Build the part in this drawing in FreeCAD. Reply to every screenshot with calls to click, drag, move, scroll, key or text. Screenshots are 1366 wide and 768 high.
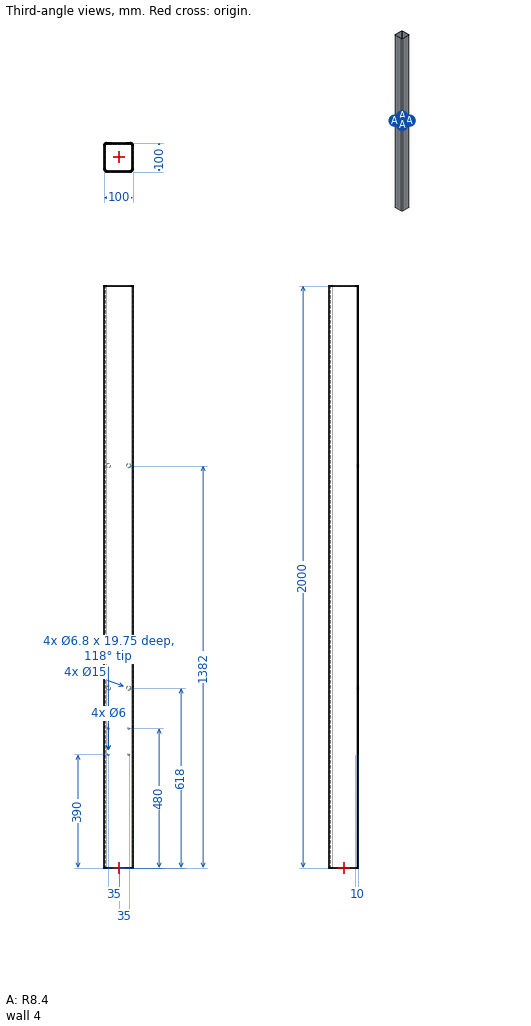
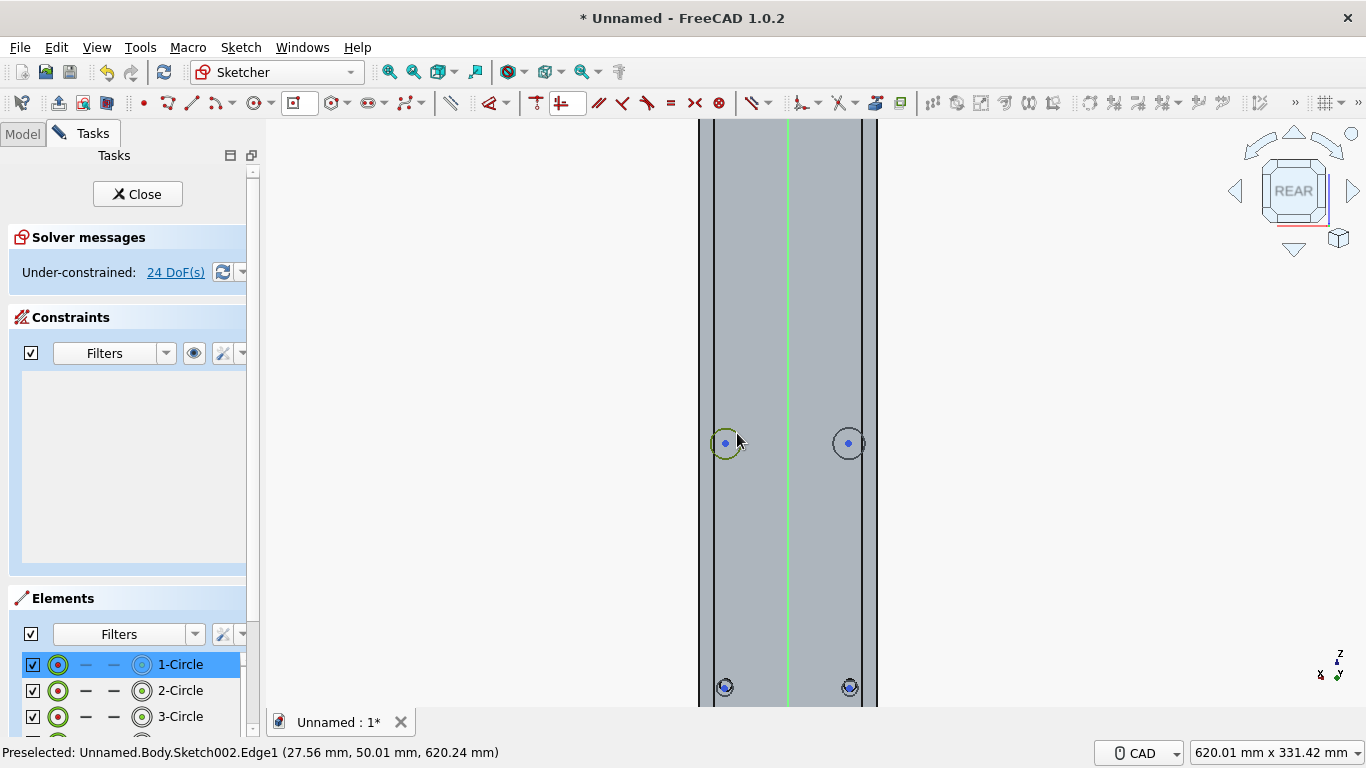
click(860, 432)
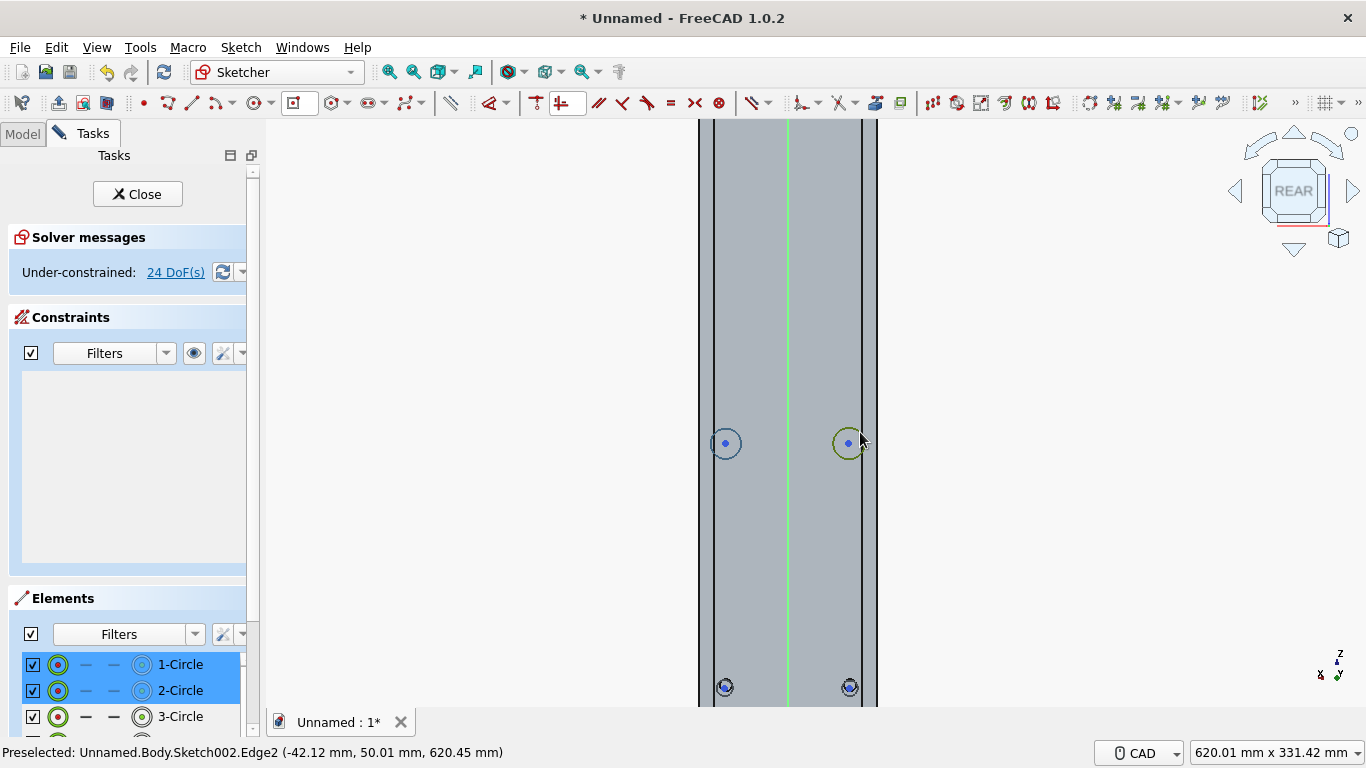
scroll(739, 435, down, 9)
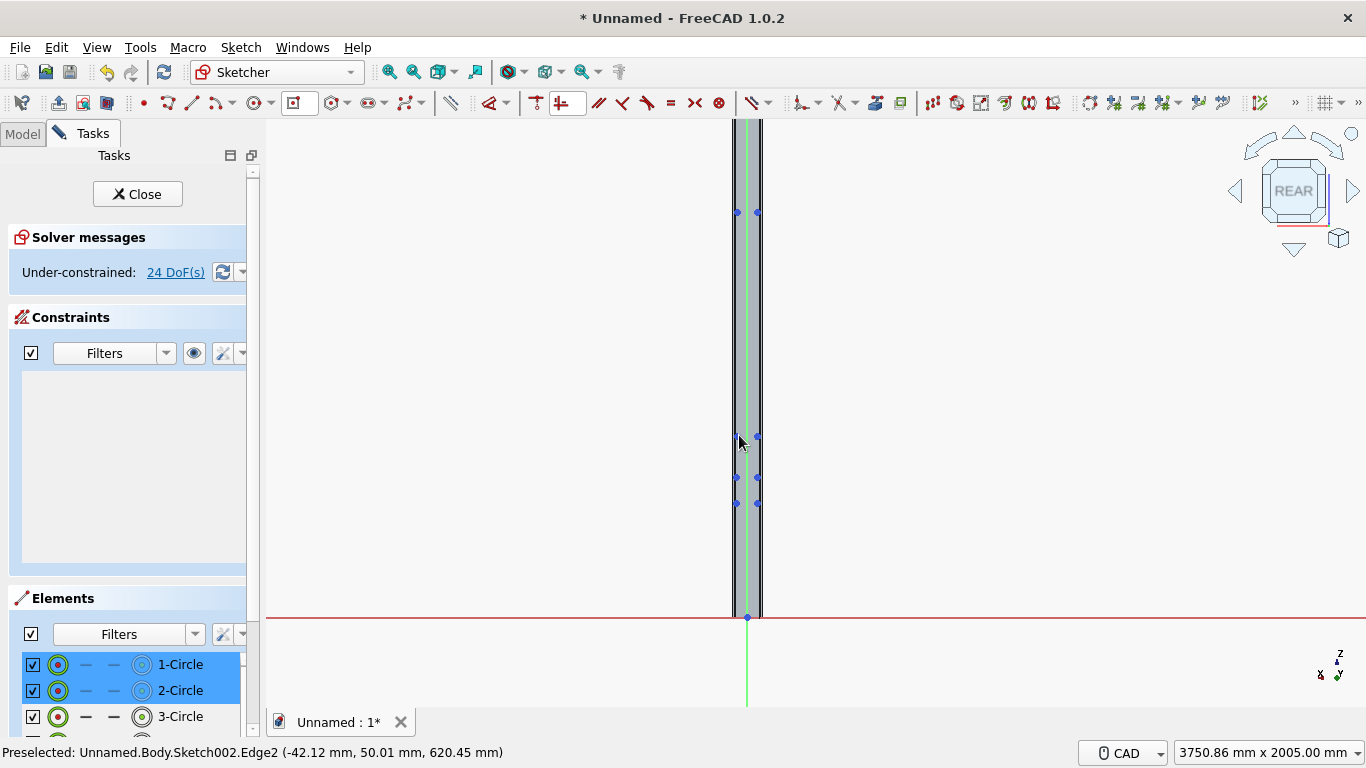
scroll(739, 211, up, 10)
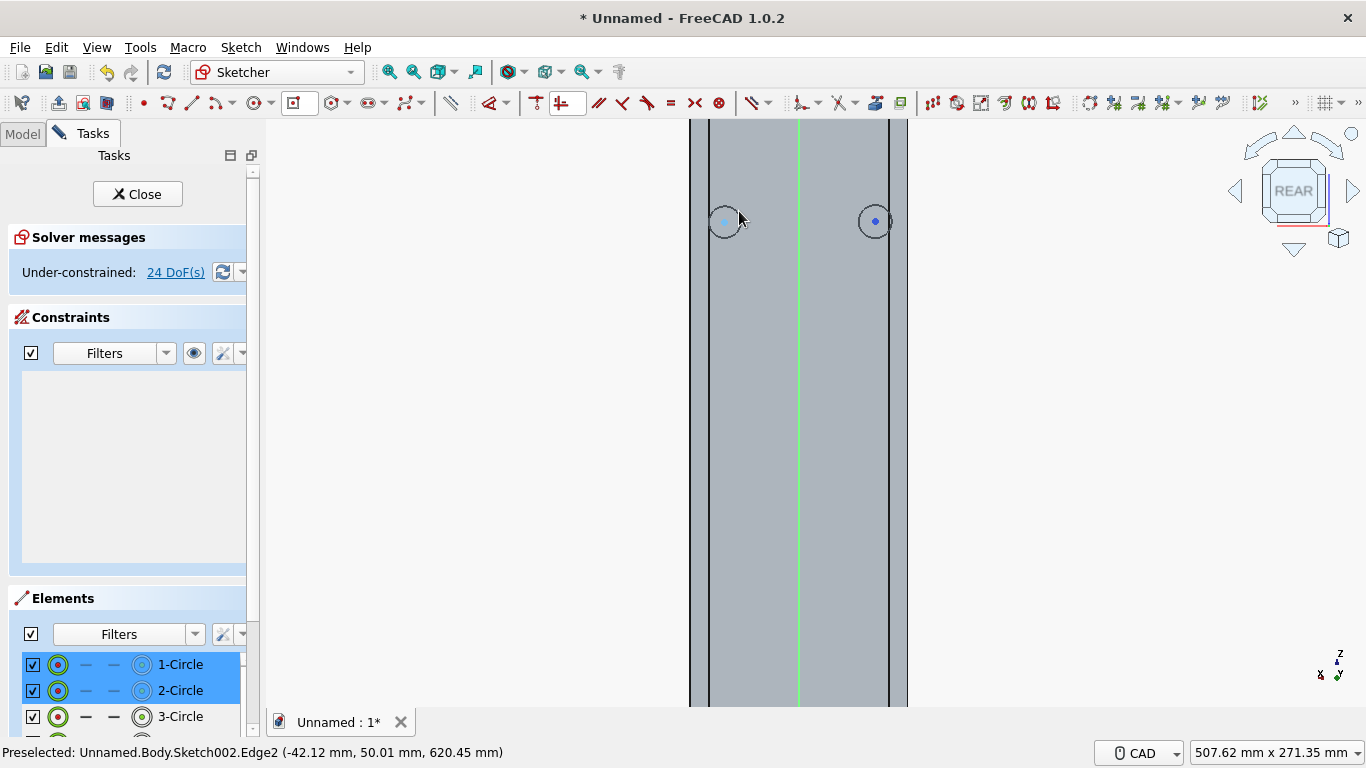
click(736, 211)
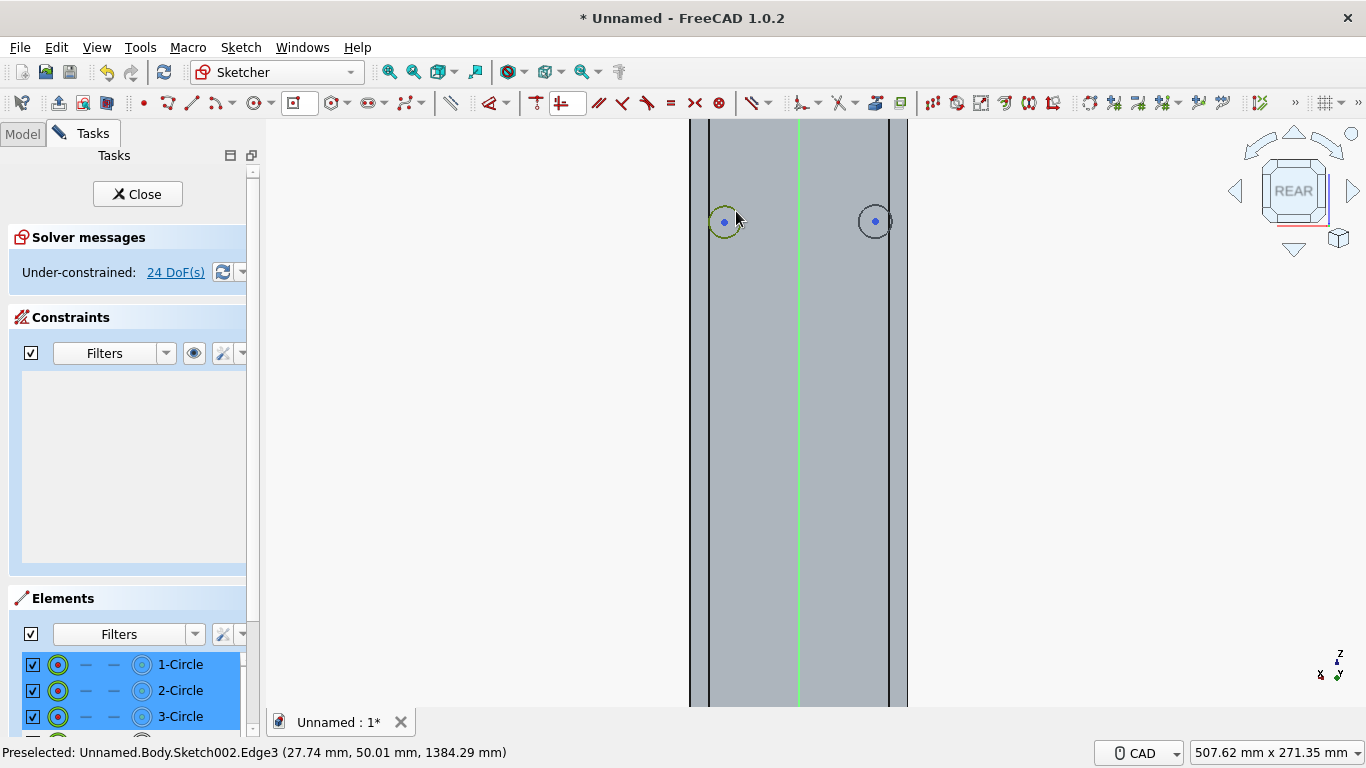
click(887, 210)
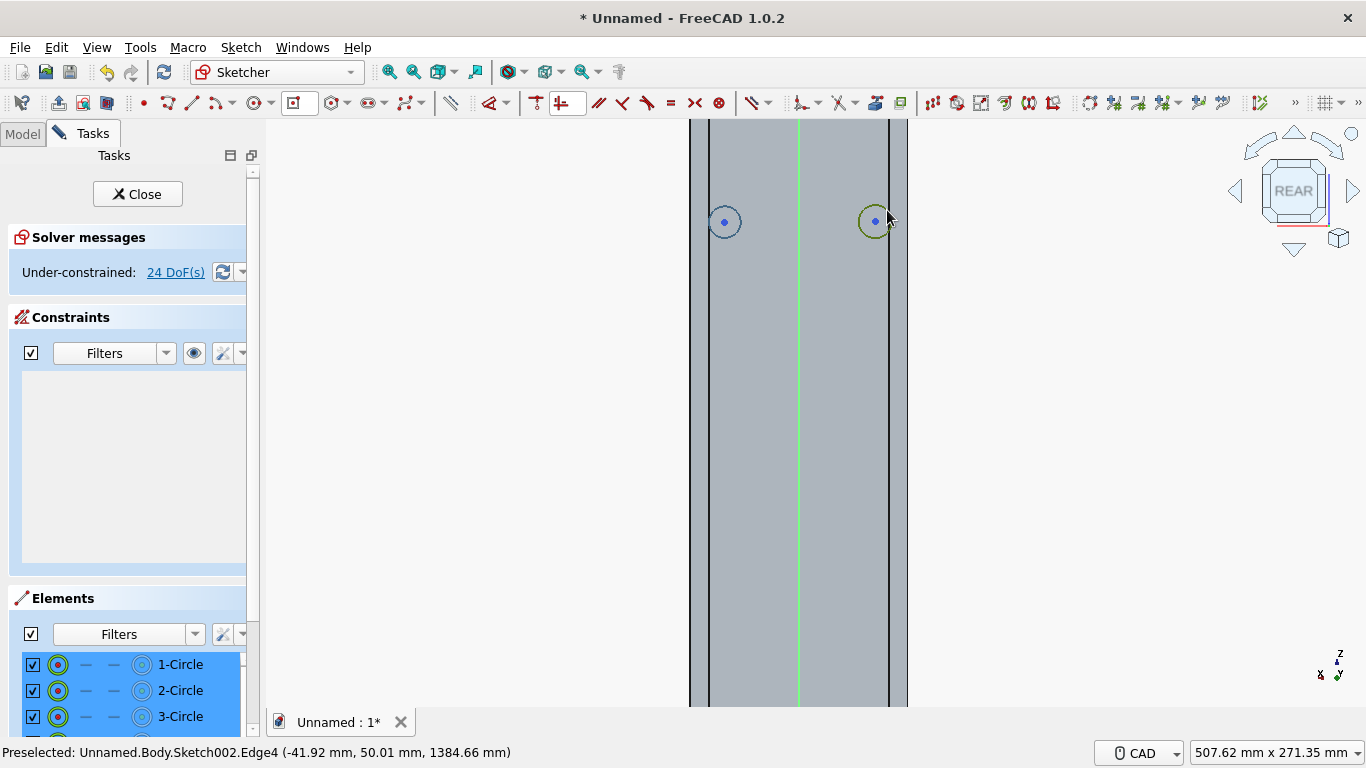
click(672, 104)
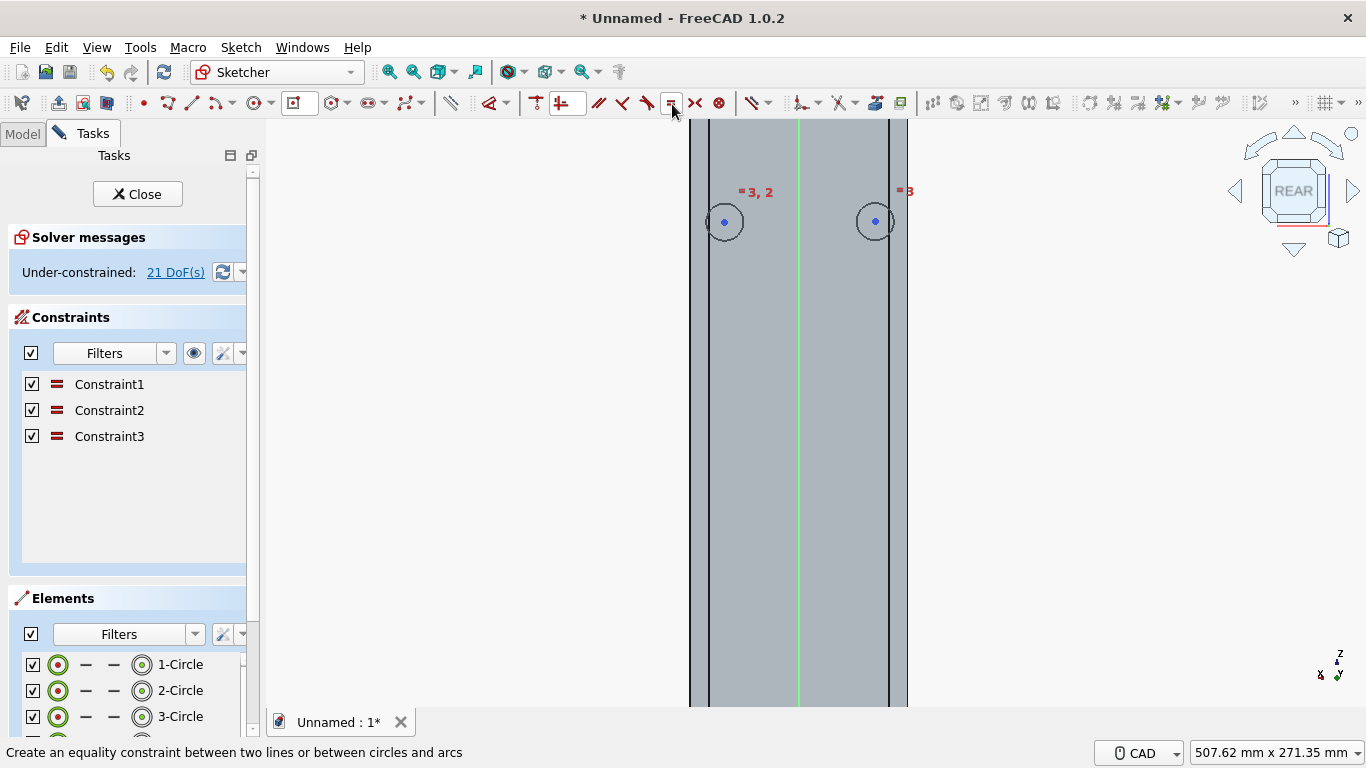
scroll(739, 210, down, 10)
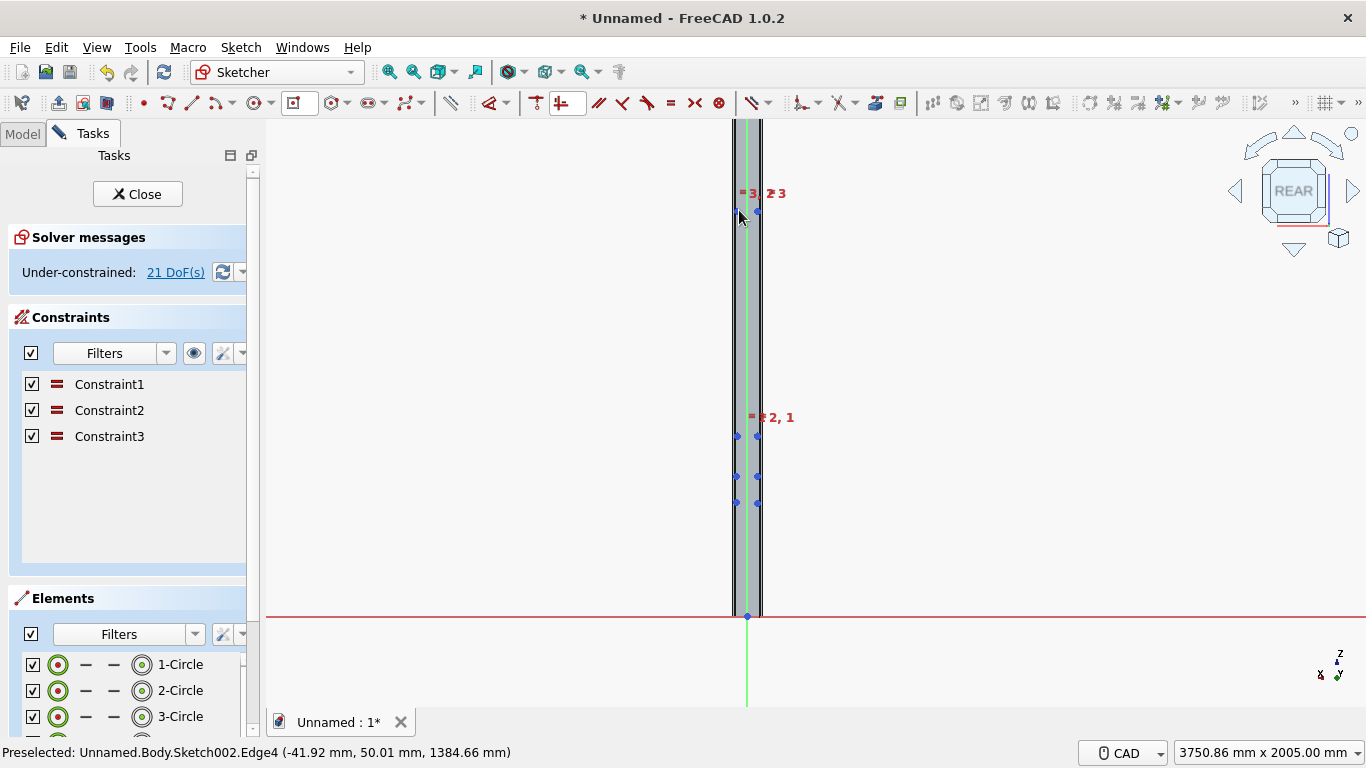
scroll(759, 502, up, 12)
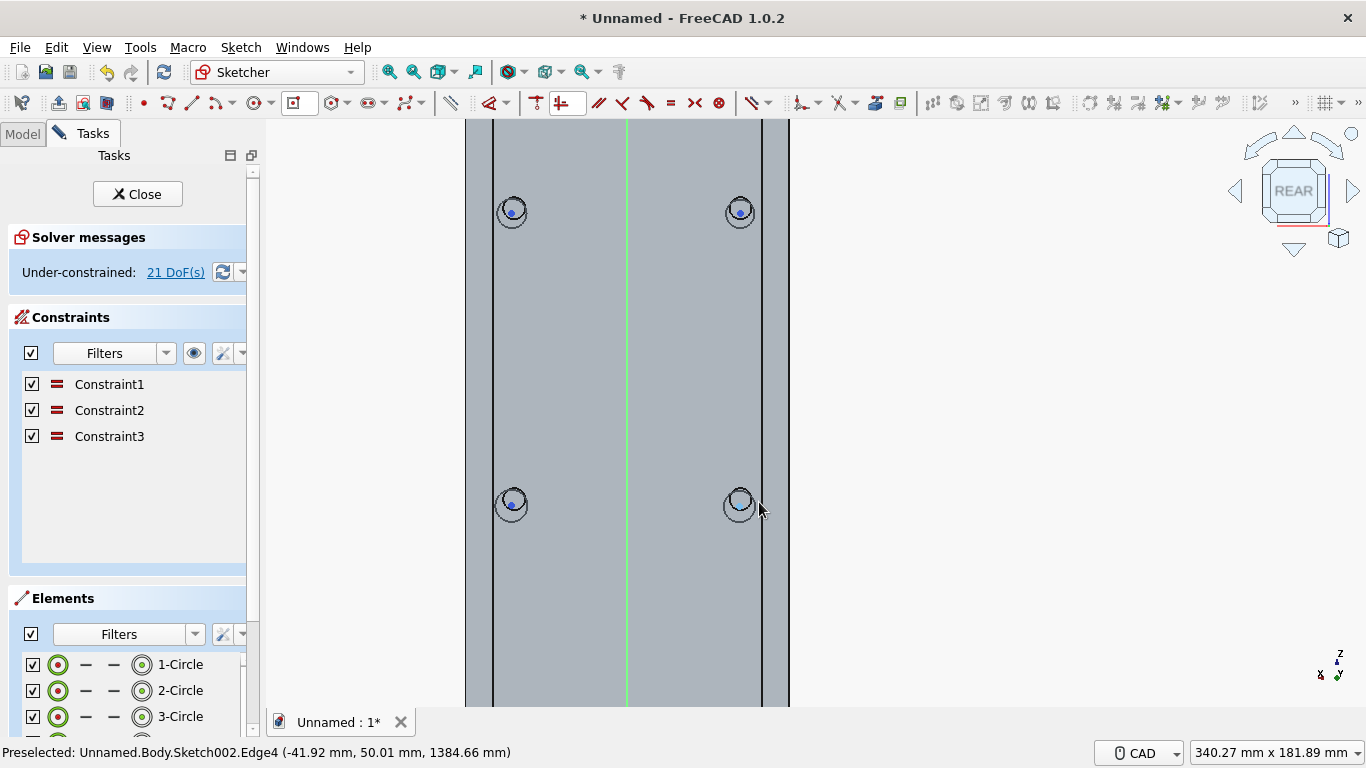
click(750, 495)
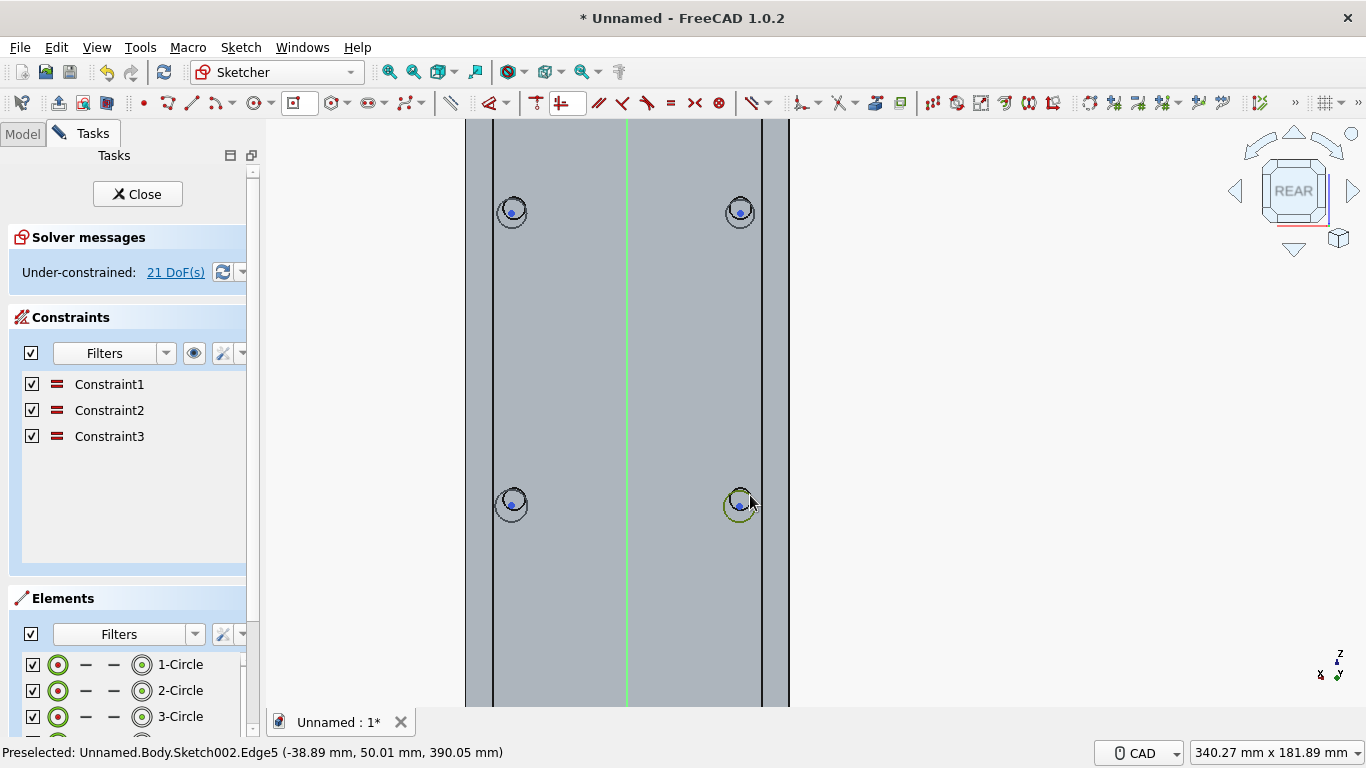
click(523, 494)